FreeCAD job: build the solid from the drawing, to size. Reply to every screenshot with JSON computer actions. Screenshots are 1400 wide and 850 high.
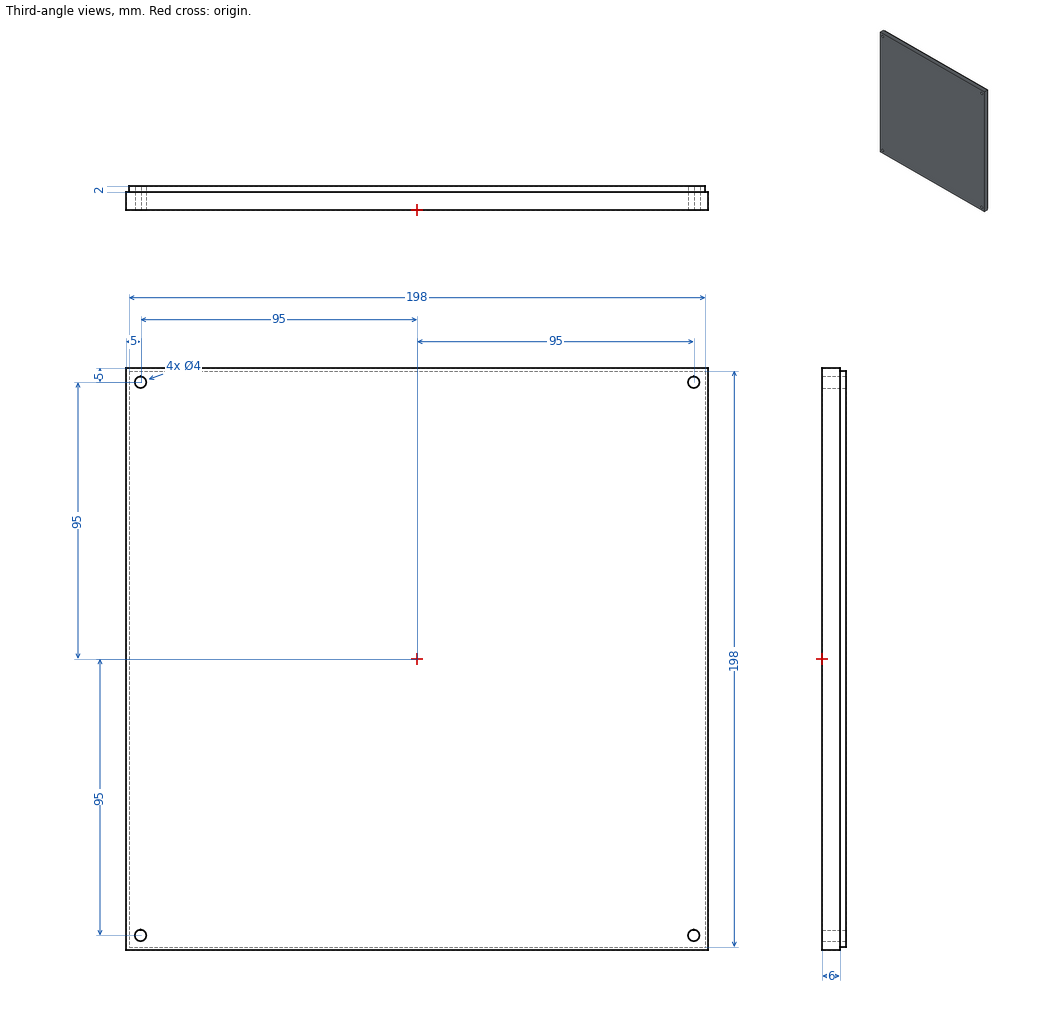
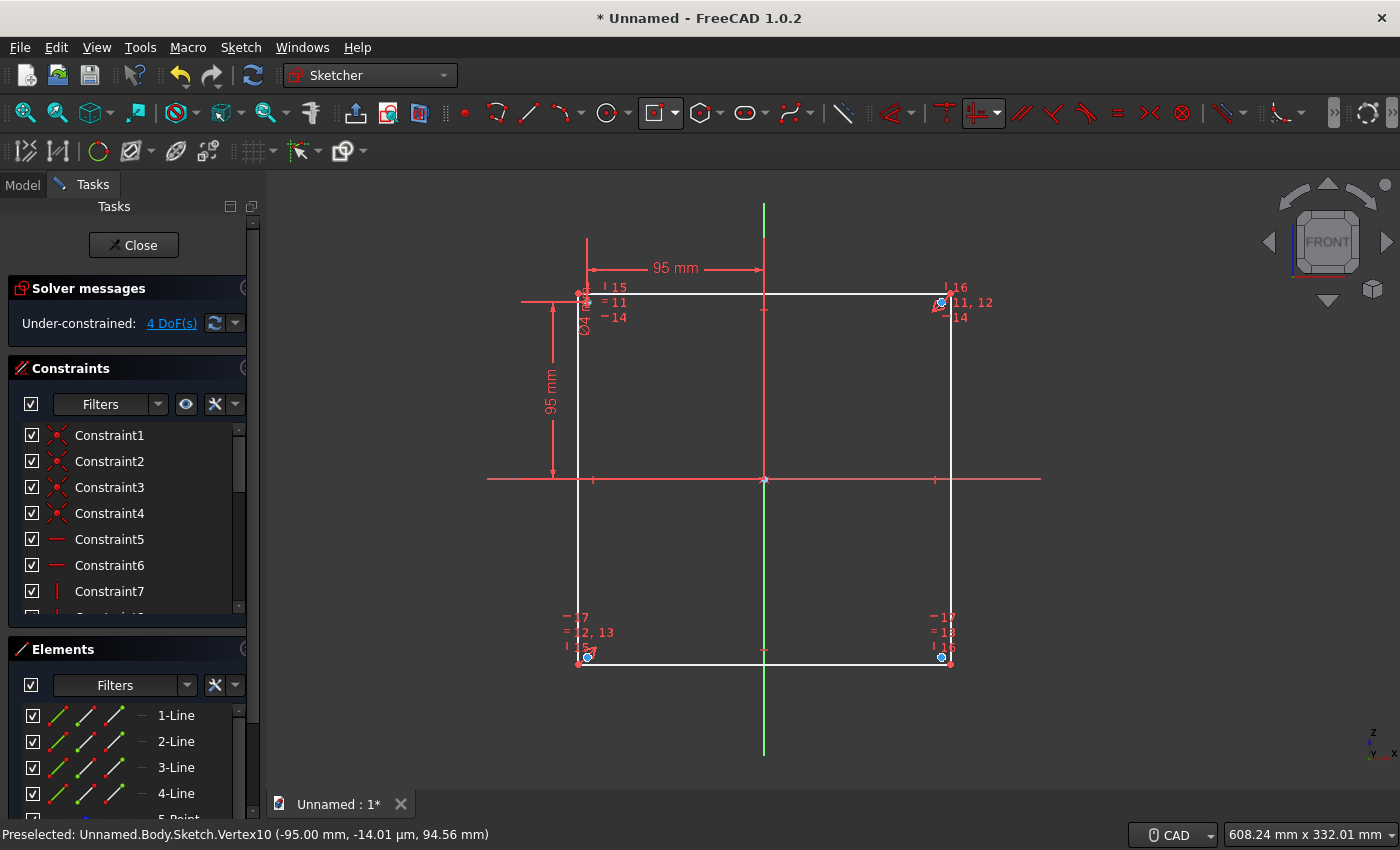
{"action": "left_click", "coordinate": [942, 302]}
{"action": "left_click", "coordinate": [853, 268]}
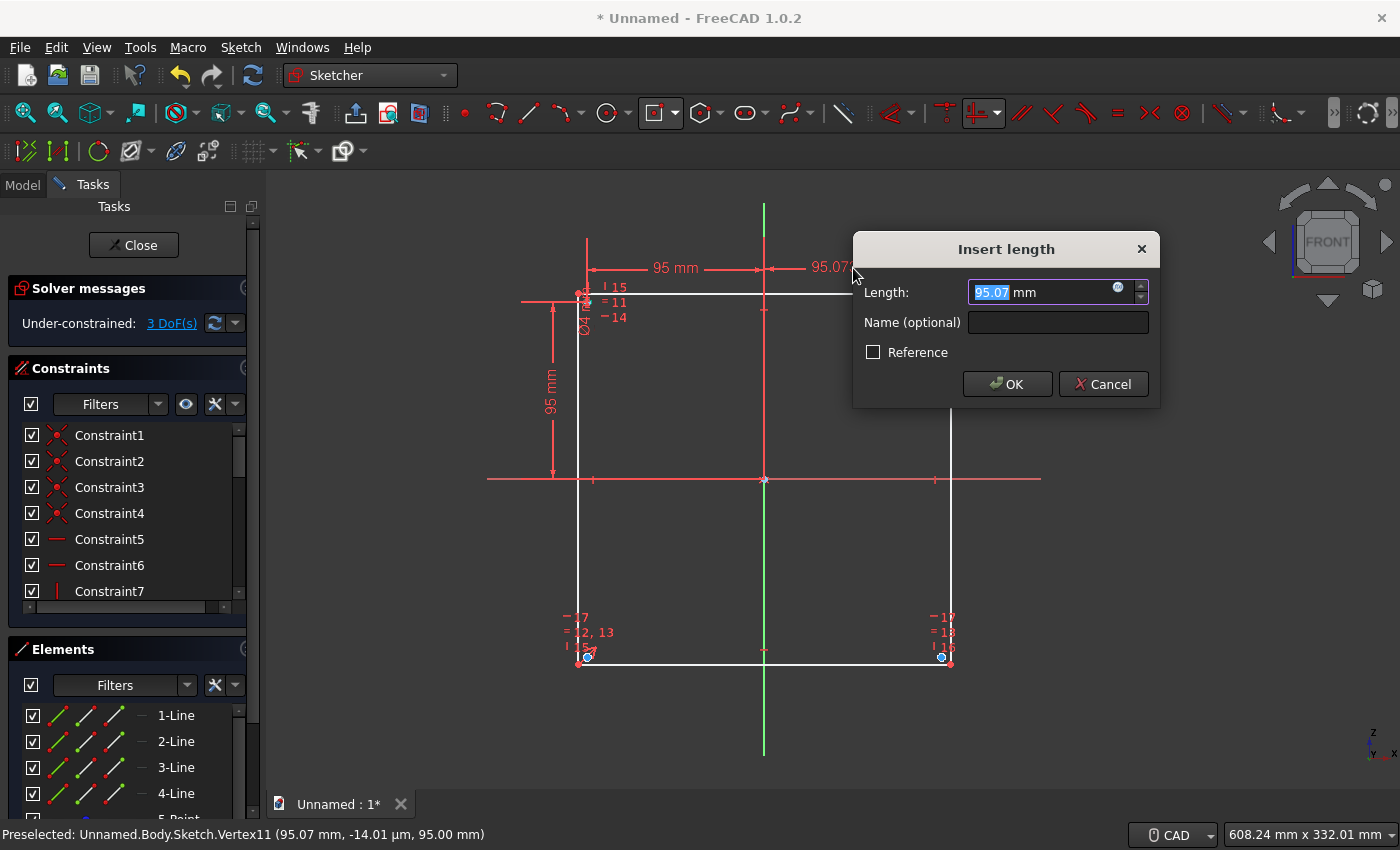
{"action": "type", "text": "95"}
{"action": "key", "text": "Return"}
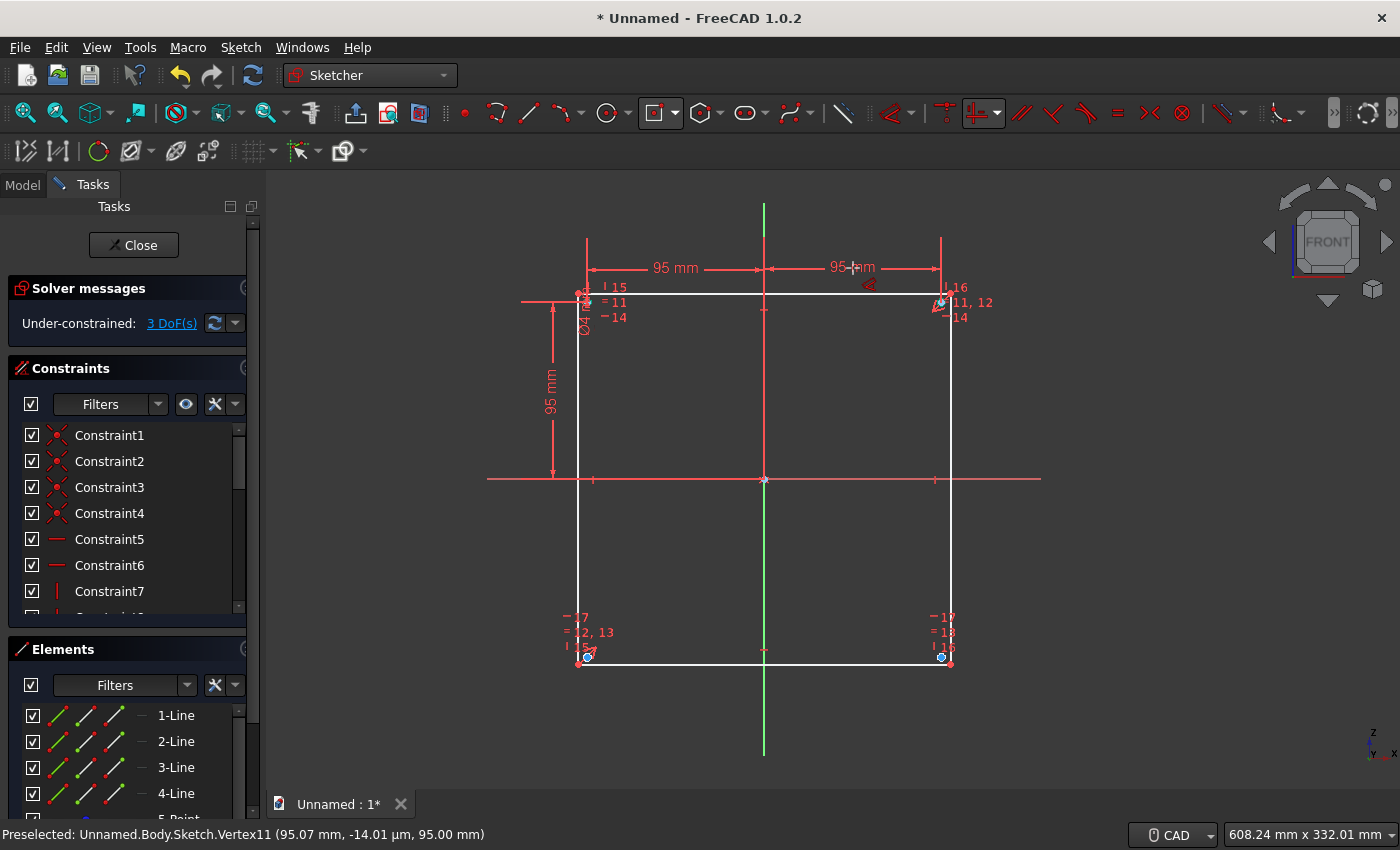
{"action": "left_click", "coordinate": [587, 657]}
{"action": "left_click", "coordinate": [553, 568]}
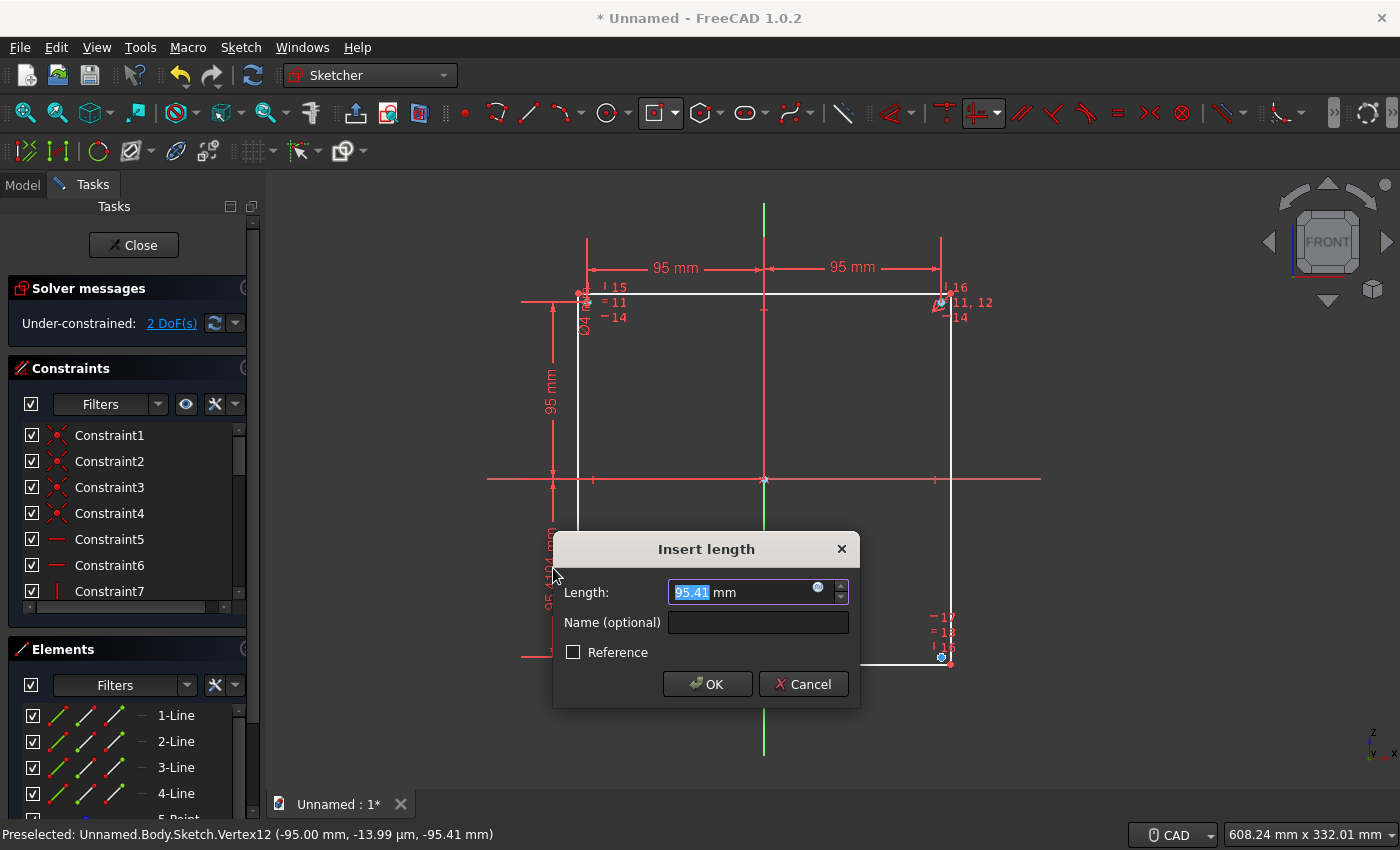
{"action": "type", "text": "95"}
{"action": "key", "text": "Return"}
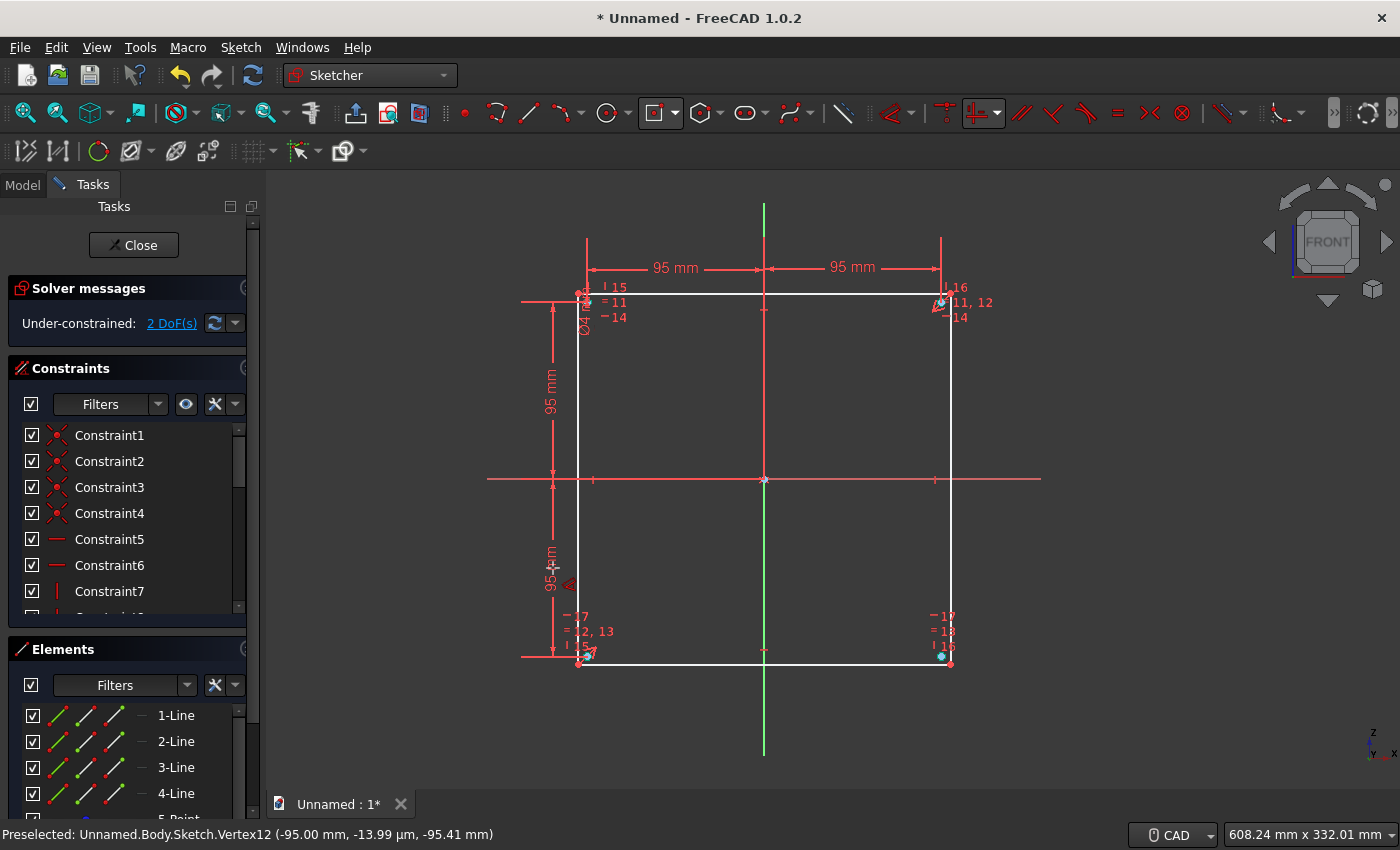
{"action": "scroll", "coordinate": [578, 294], "scroll_direction": "up", "scroll_amount": 8}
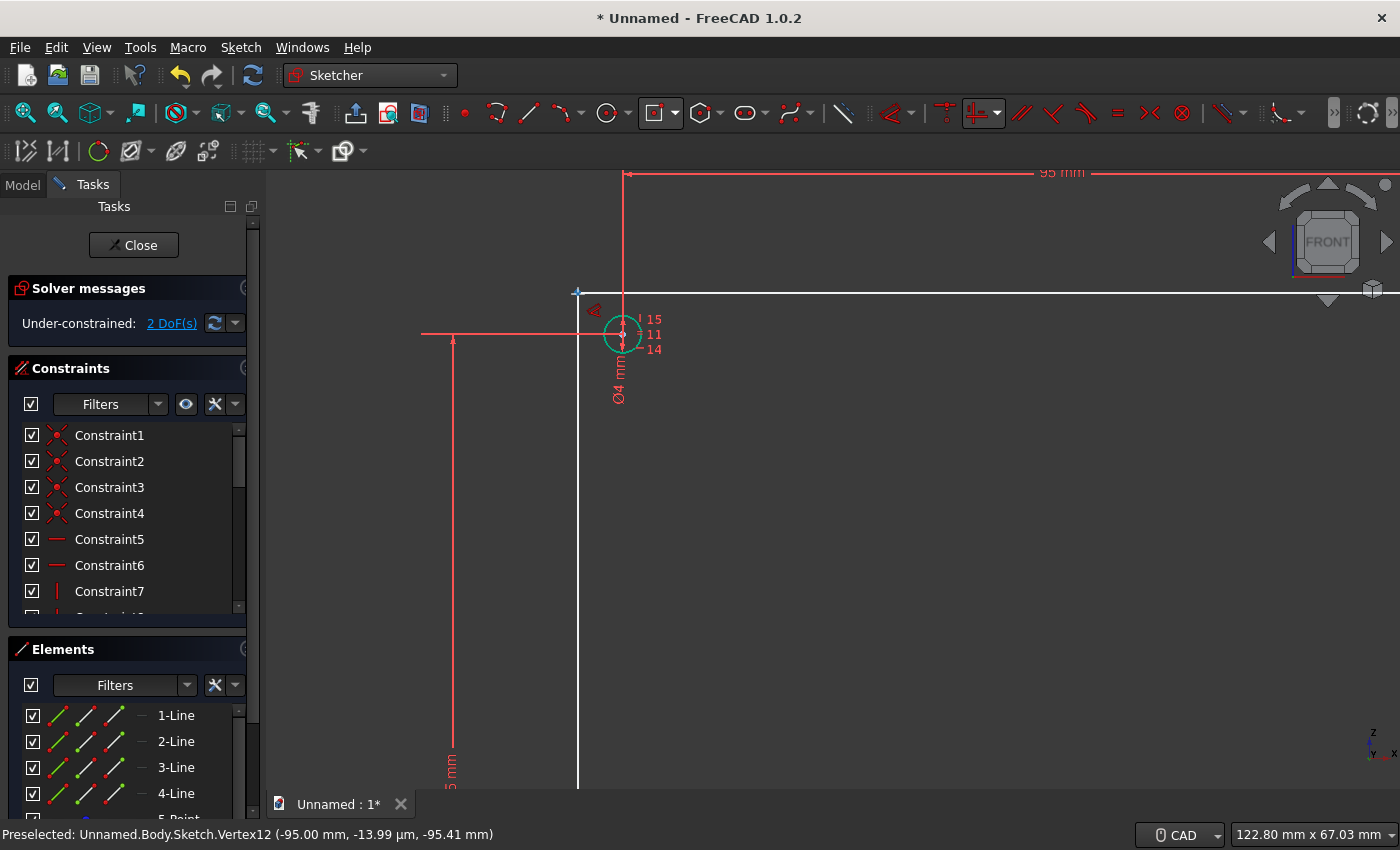
{"action": "left_click", "coordinate": [578, 293]}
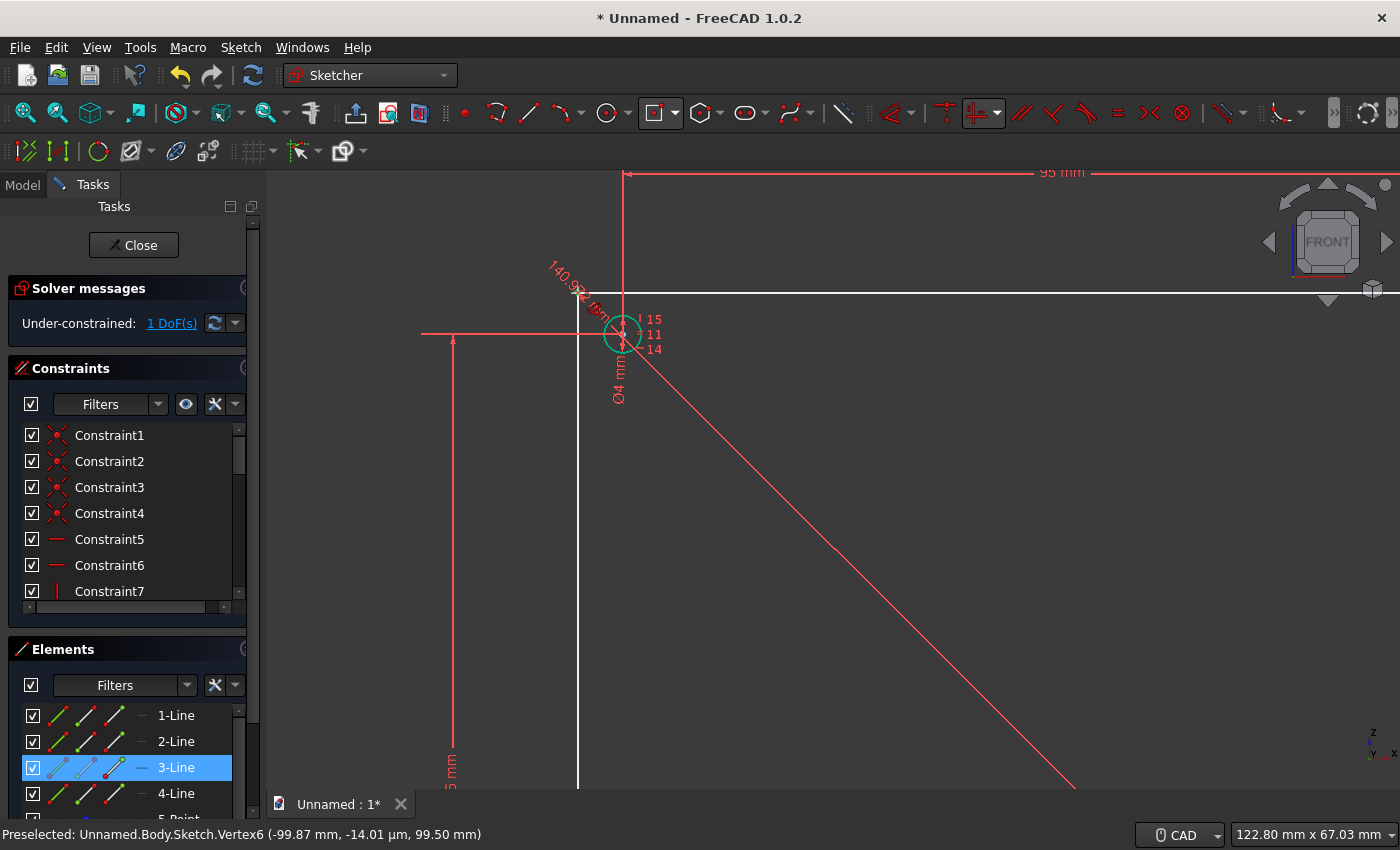
{"action": "left_click", "coordinate": [623, 334]}
{"action": "left_click", "coordinate": [600, 259]}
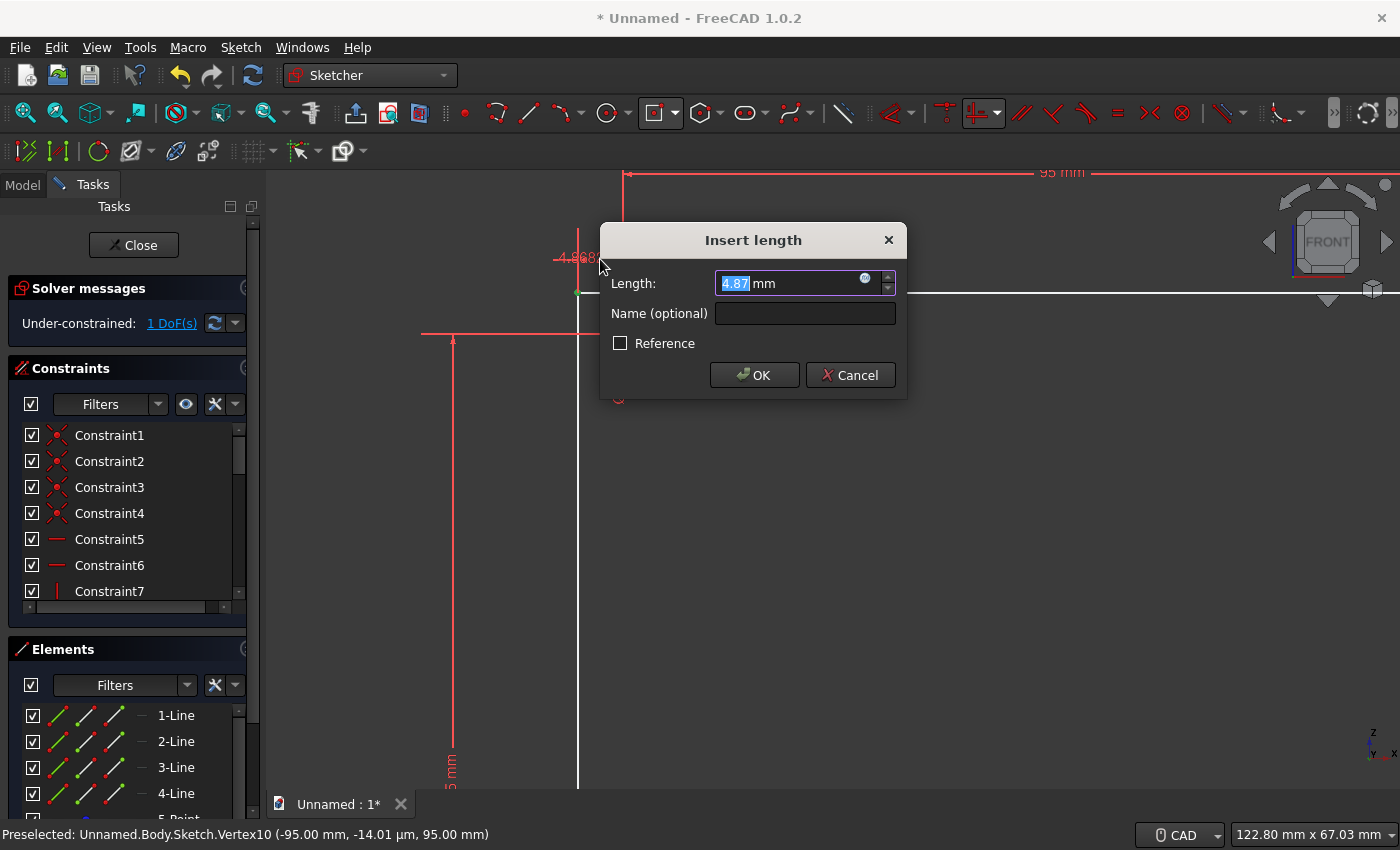
{"action": "type", "text": "5"}
{"action": "key", "text": "Return"}